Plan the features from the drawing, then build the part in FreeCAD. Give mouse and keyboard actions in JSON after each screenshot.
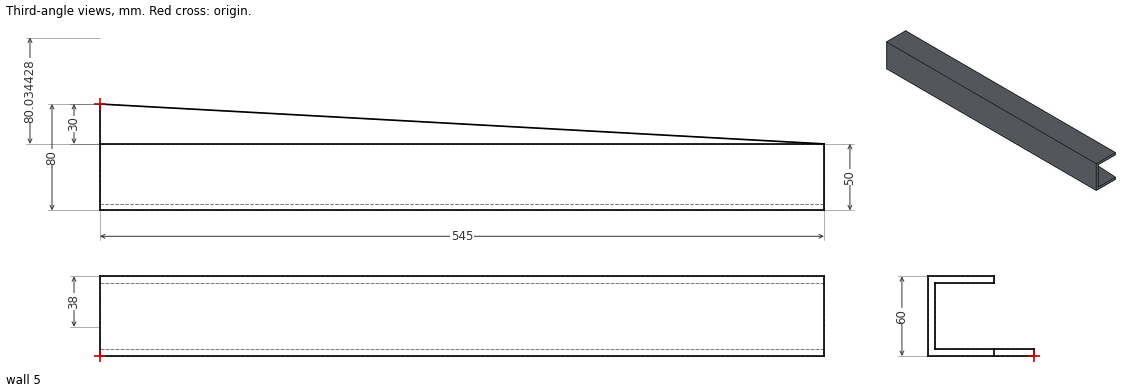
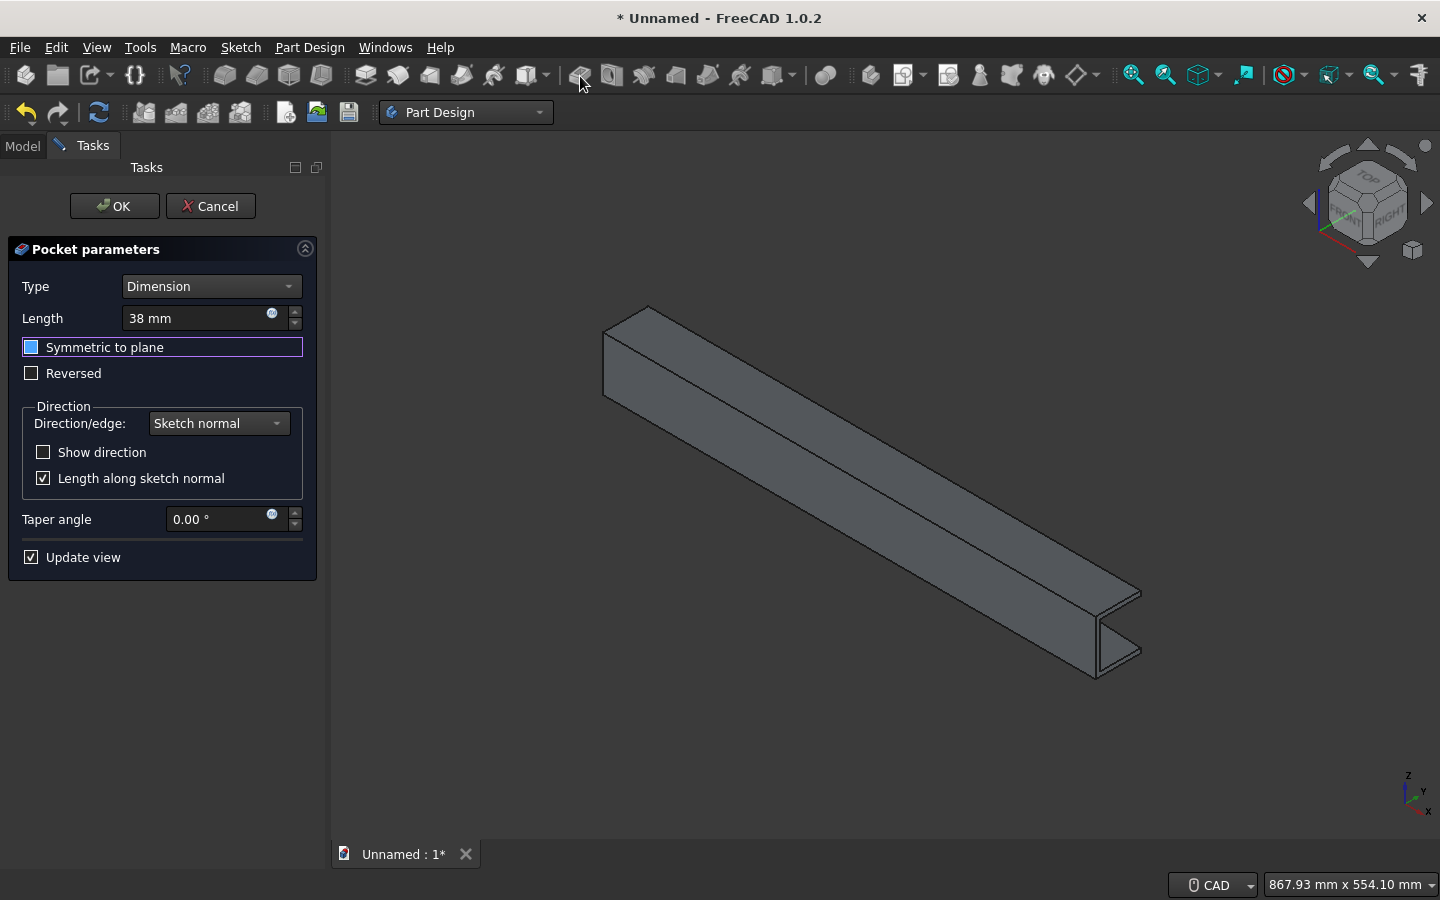
{"action": "left_click", "coordinate": [115, 206]}